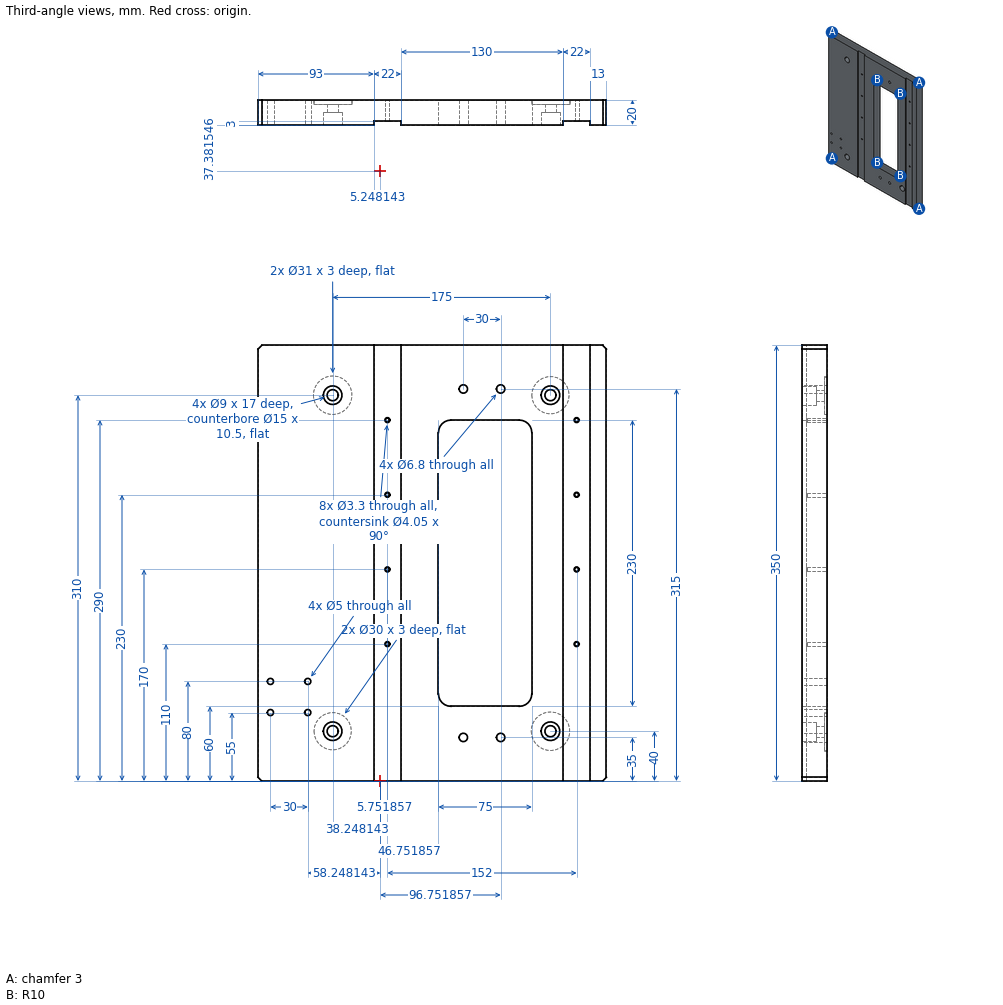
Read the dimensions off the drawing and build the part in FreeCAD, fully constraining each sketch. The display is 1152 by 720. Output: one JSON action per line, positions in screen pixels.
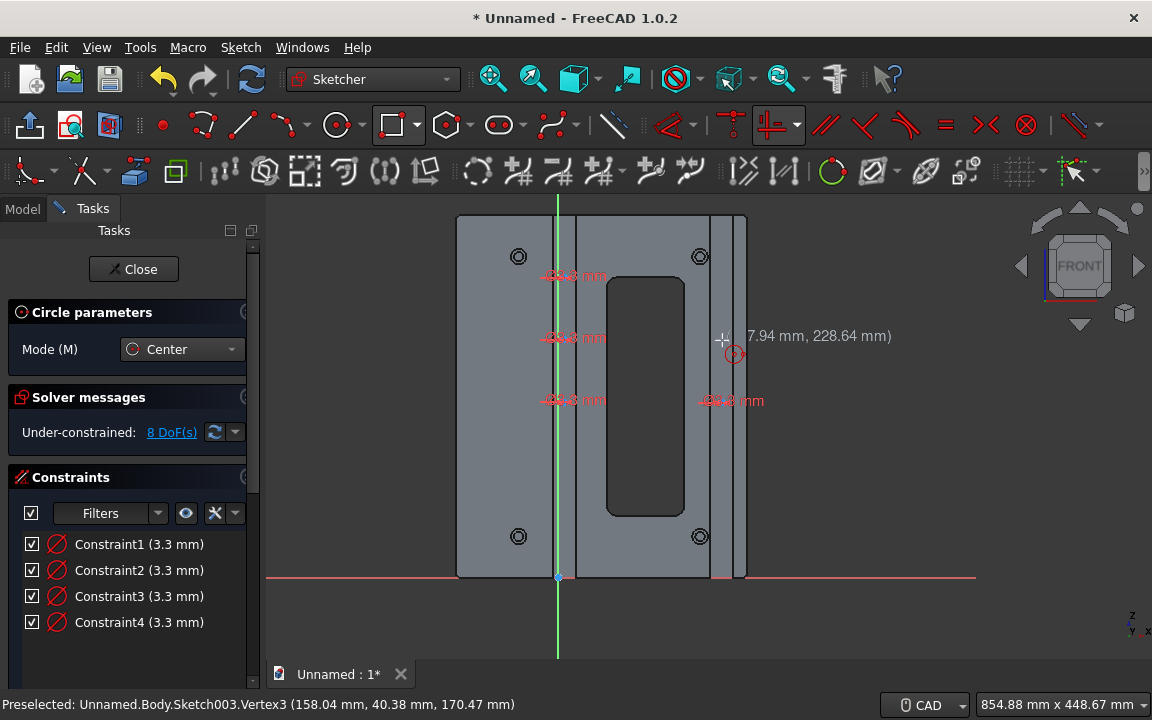
{"action": "left_click", "coordinate": [722, 340]}
{"action": "mouse_move", "coordinate": [723, 338]}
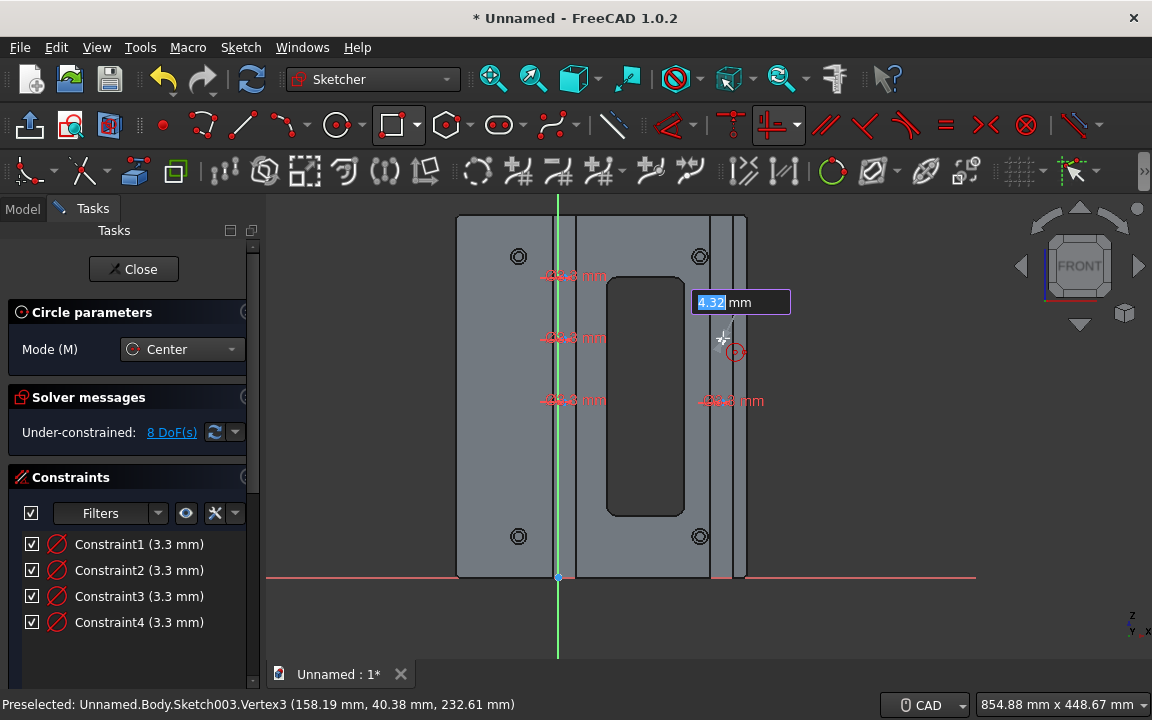
{"action": "type", "text": "3.3"}
{"action": "key", "text": "Return"}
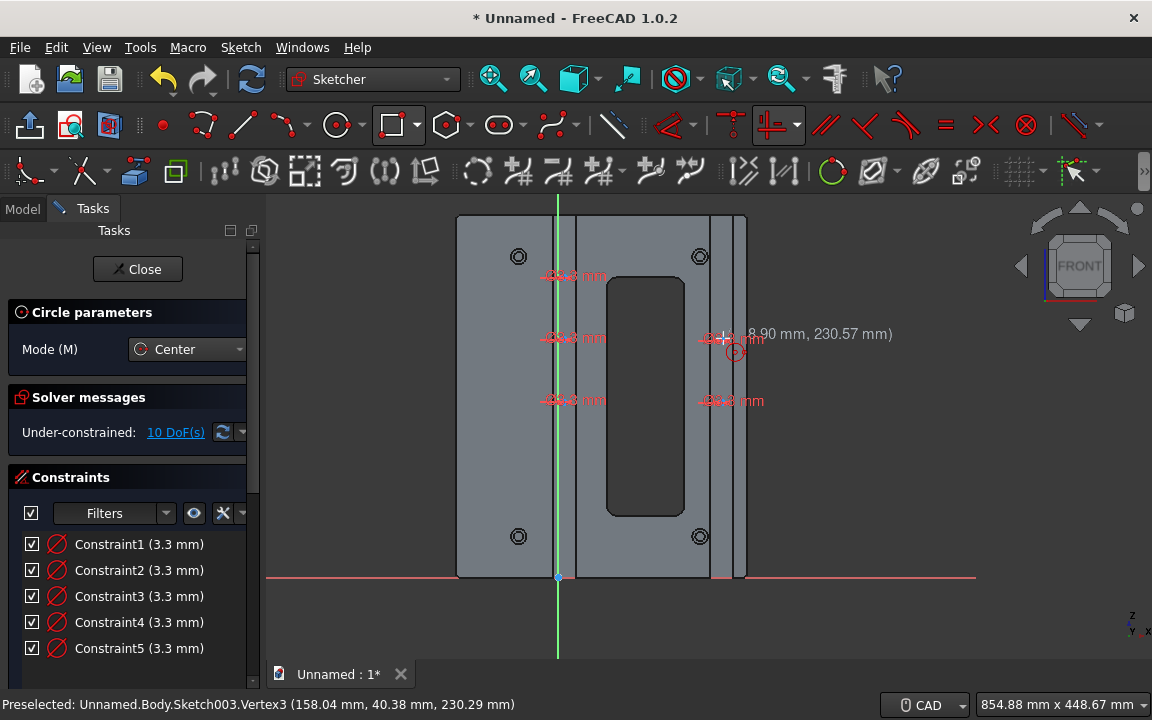
{"action": "scroll", "coordinate": [722, 277], "scroll_direction": "up", "scroll_amount": 13}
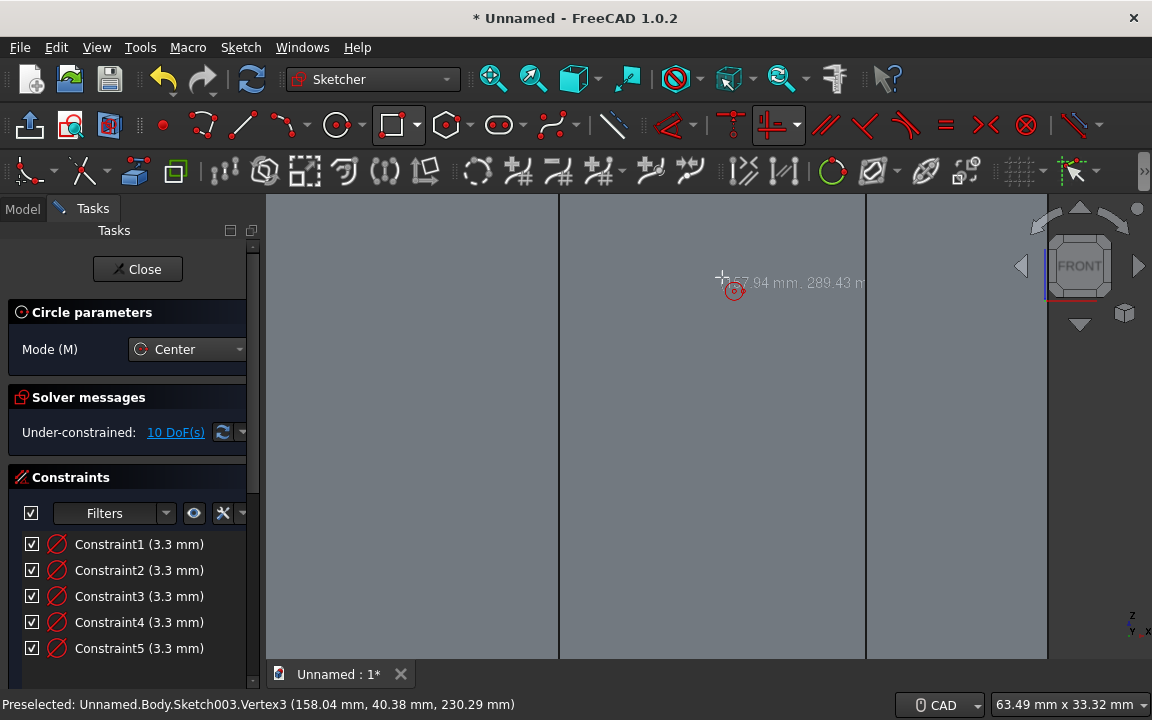
{"action": "scroll", "coordinate": [722, 277], "scroll_direction": "down", "scroll_amount": 13}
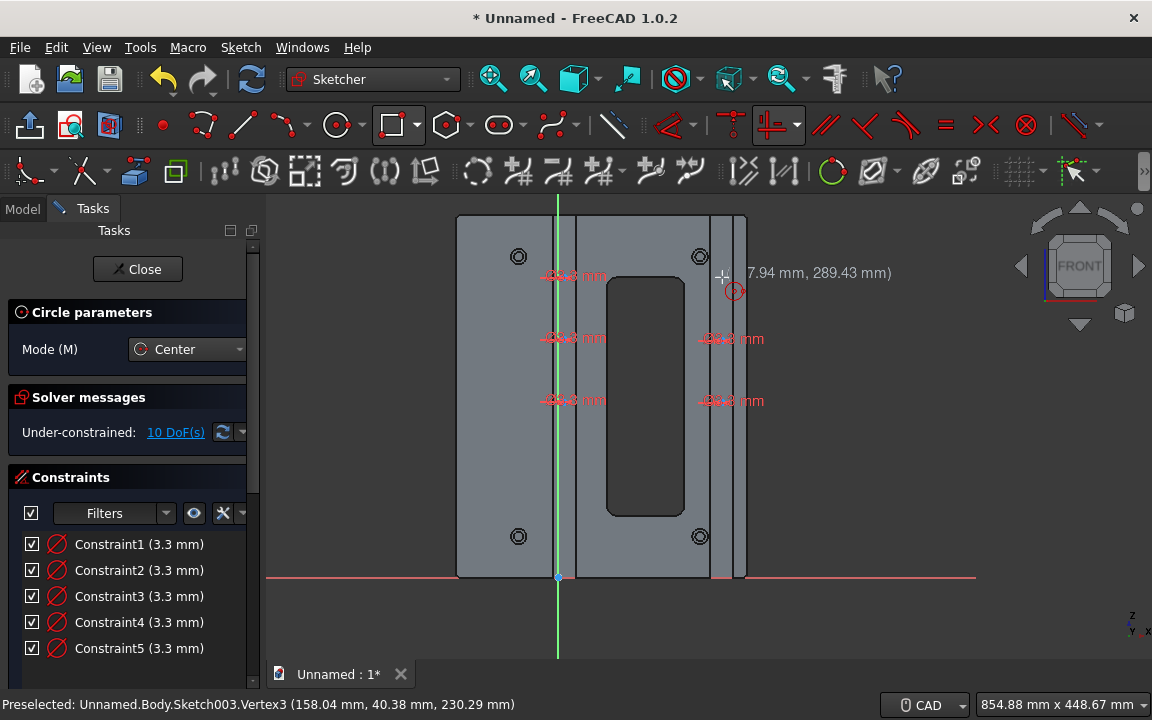
{"action": "left_click", "coordinate": [722, 277]}
{"action": "mouse_move", "coordinate": [723, 276]}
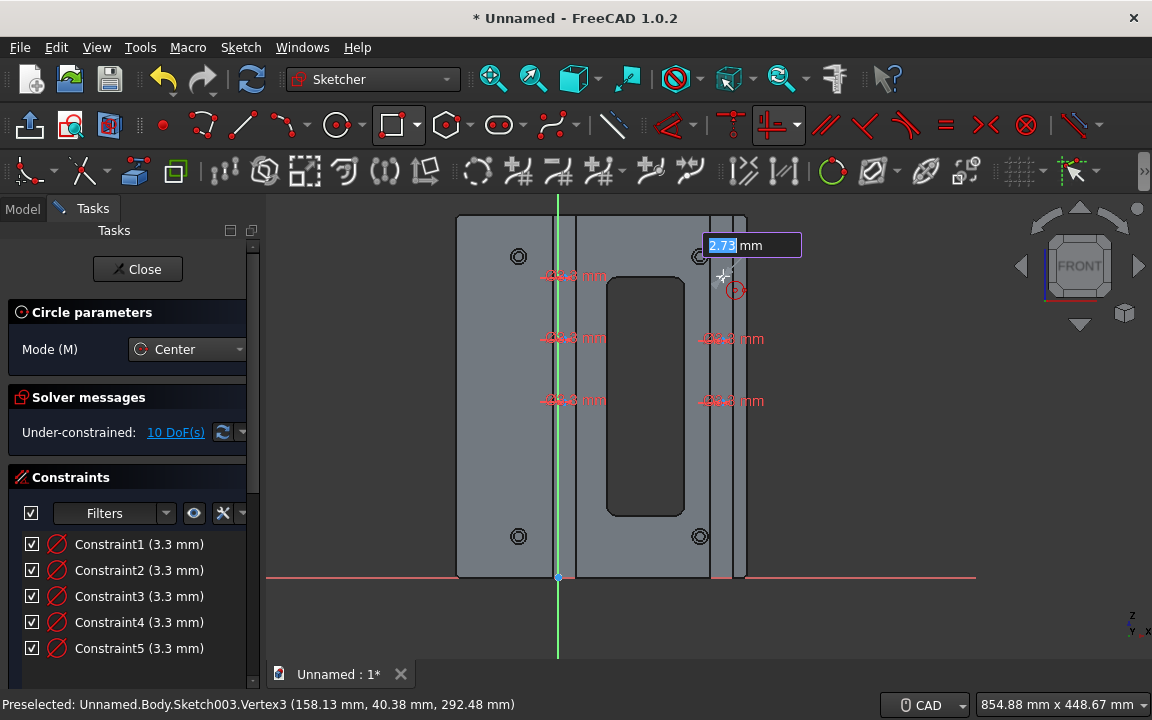
{"action": "type", "text": "3.3"}
{"action": "key", "text": "Return"}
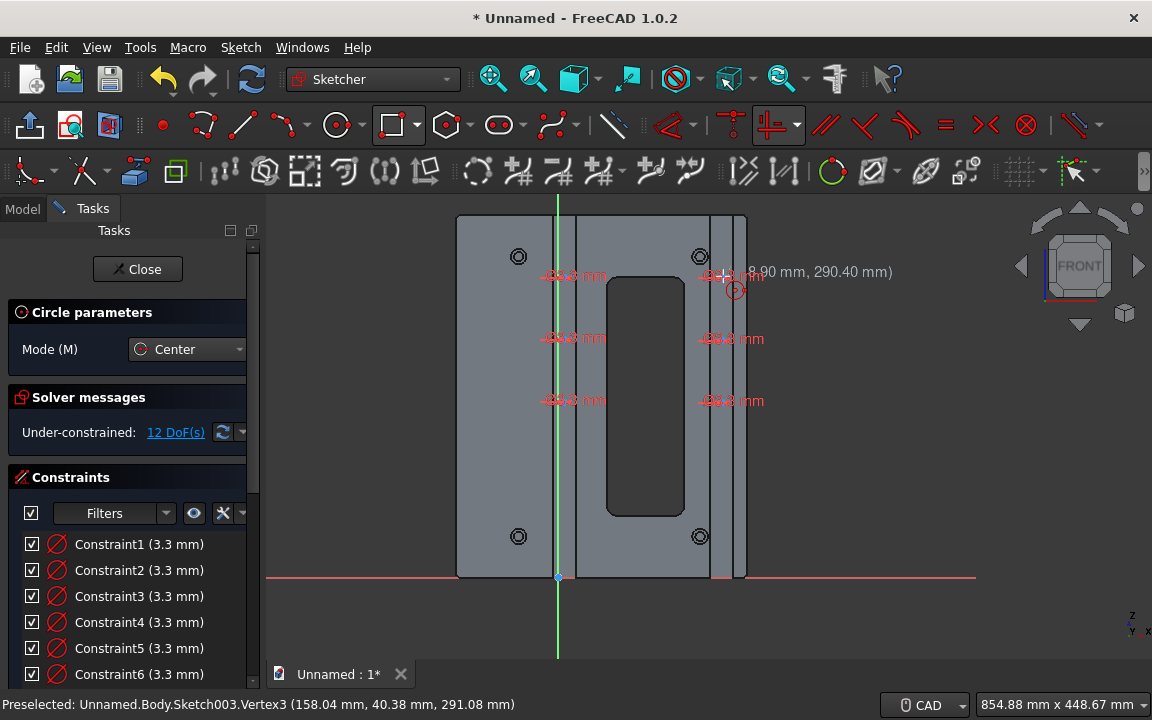
{"action": "scroll", "coordinate": [564, 464], "scroll_direction": "up", "scroll_amount": 13}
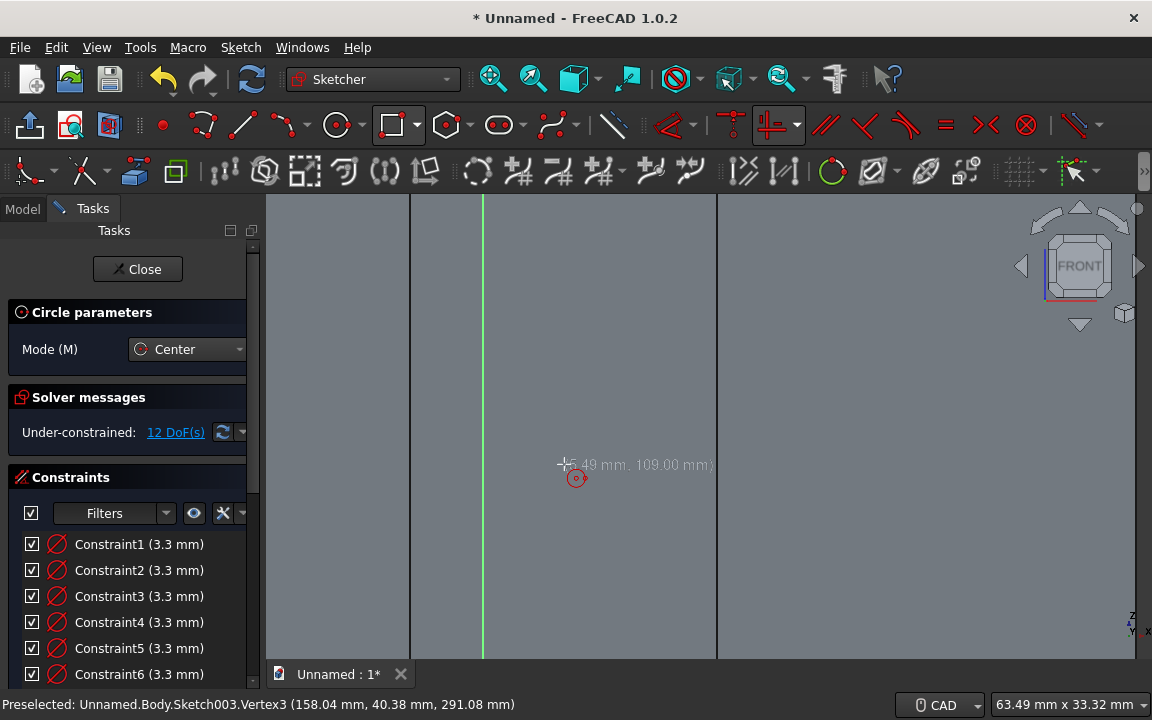
{"action": "scroll", "coordinate": [564, 464], "scroll_direction": "down", "scroll_amount": 13}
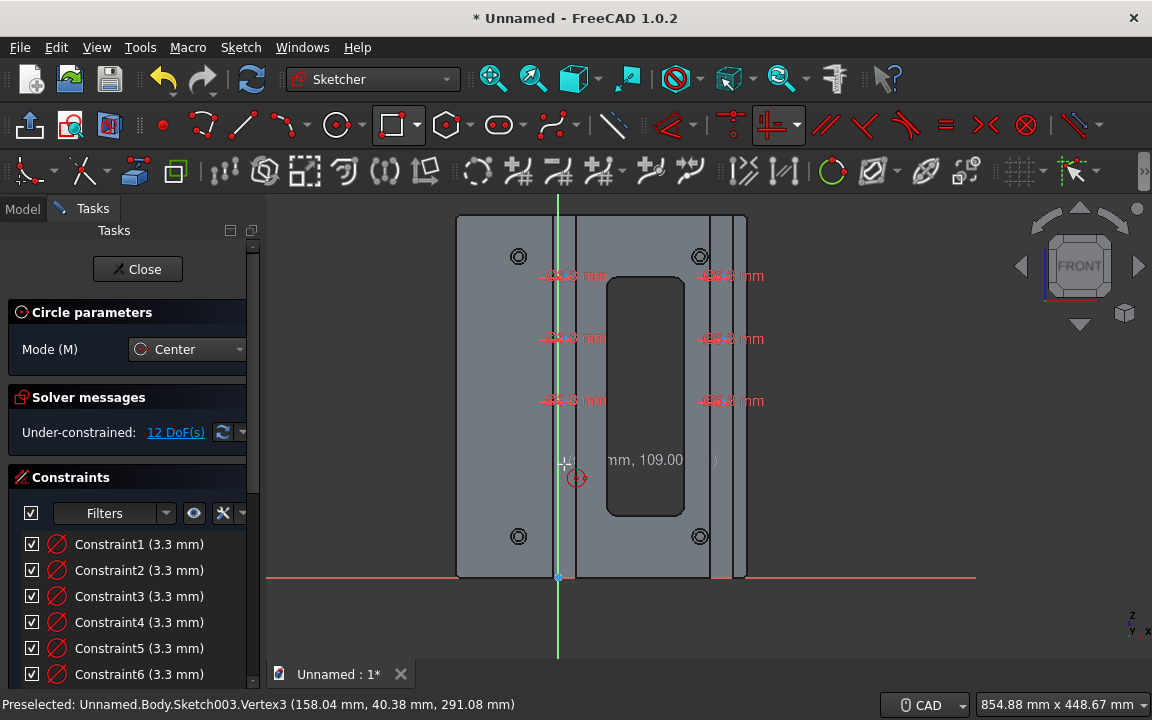
{"action": "scroll", "coordinate": [564, 464], "scroll_direction": "up", "scroll_amount": 5}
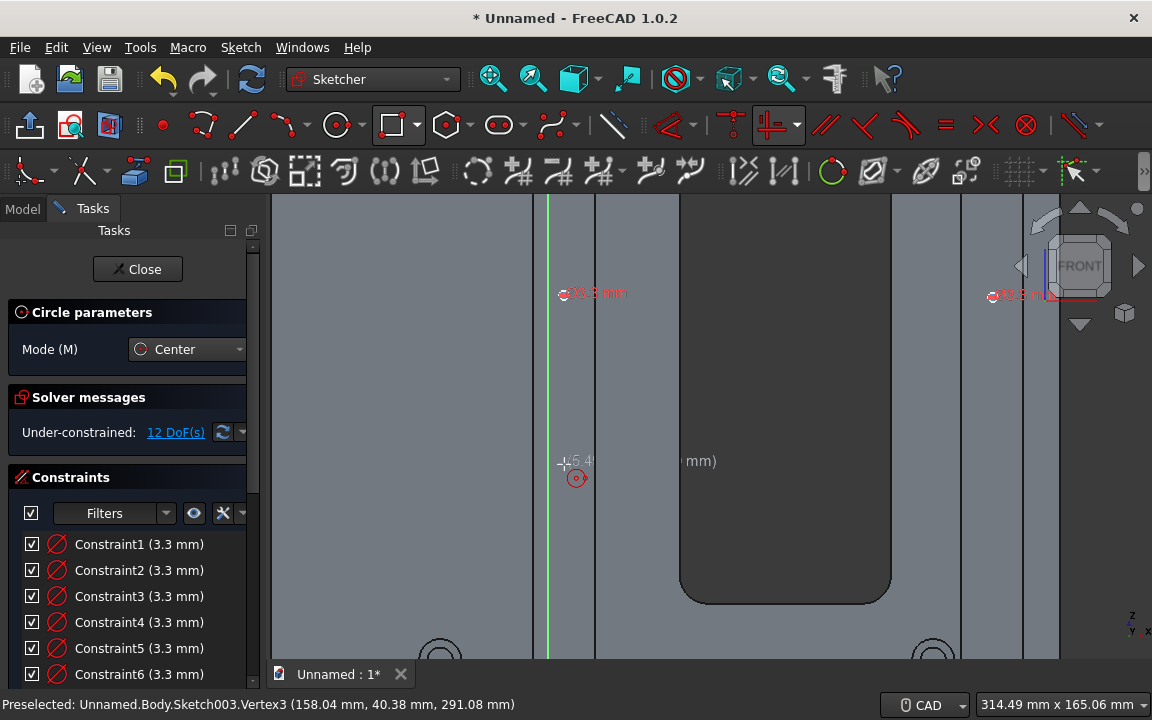
{"action": "left_click", "coordinate": [564, 463]}
{"action": "mouse_move", "coordinate": [567, 460]}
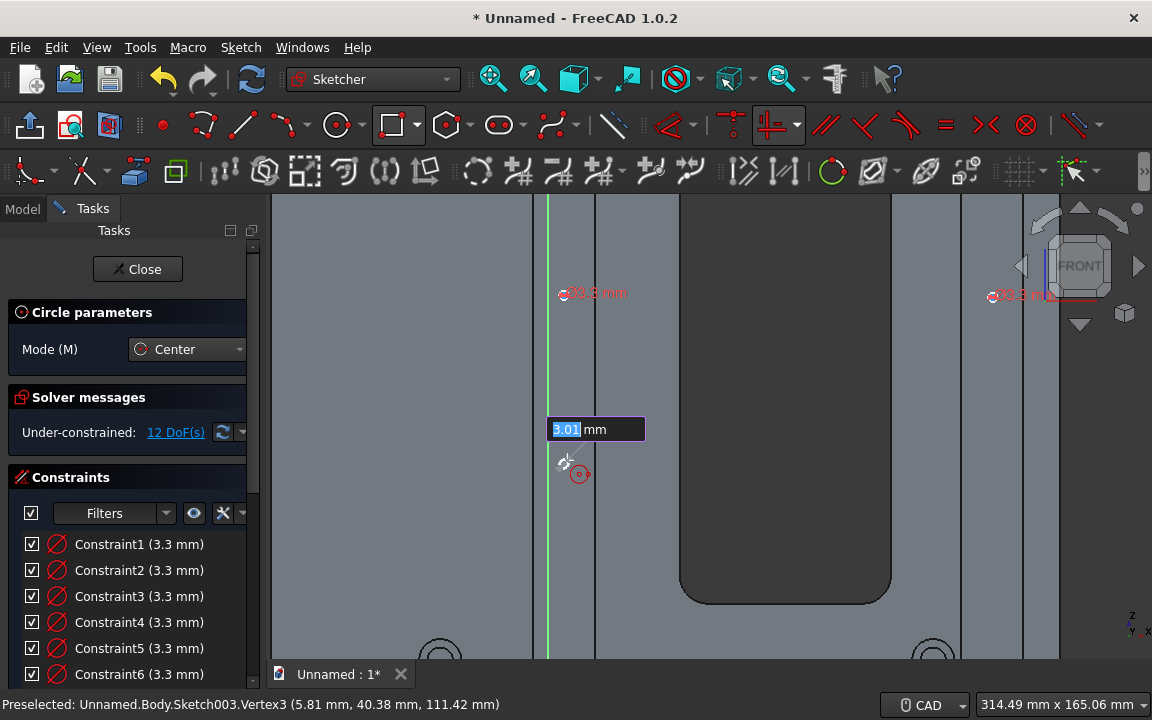
{"action": "type", "text": "3.3"}
{"action": "key", "text": "Return"}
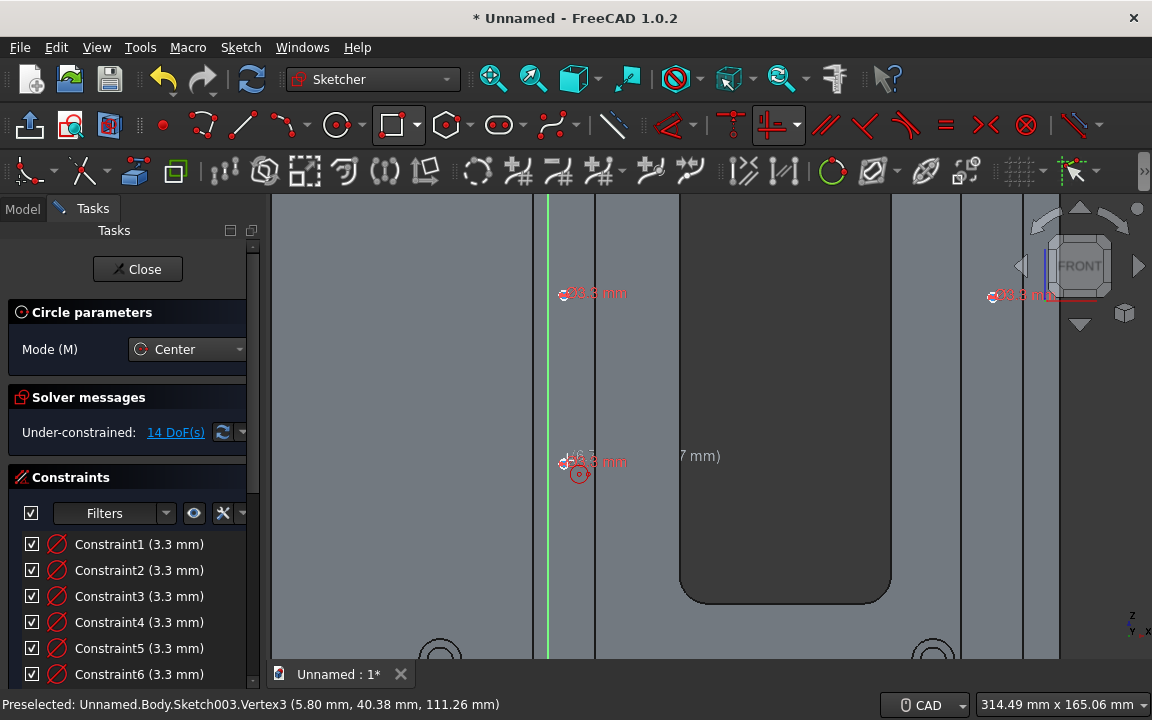
{"action": "scroll", "coordinate": [564, 464], "scroll_direction": "down", "scroll_amount": 5}